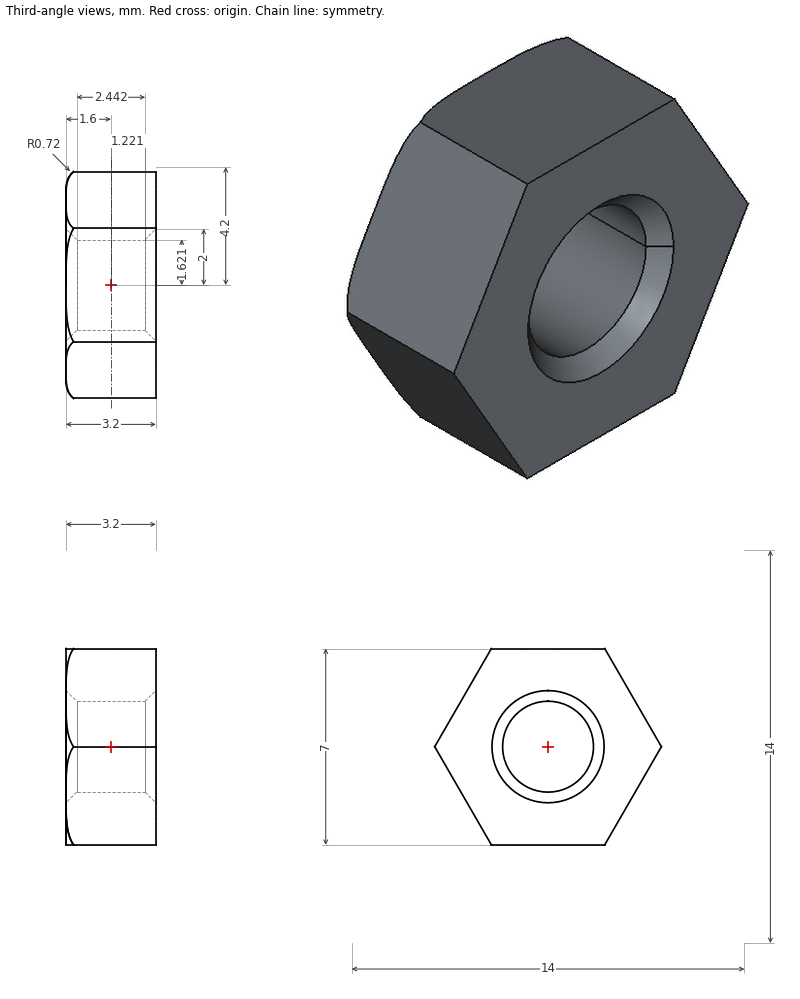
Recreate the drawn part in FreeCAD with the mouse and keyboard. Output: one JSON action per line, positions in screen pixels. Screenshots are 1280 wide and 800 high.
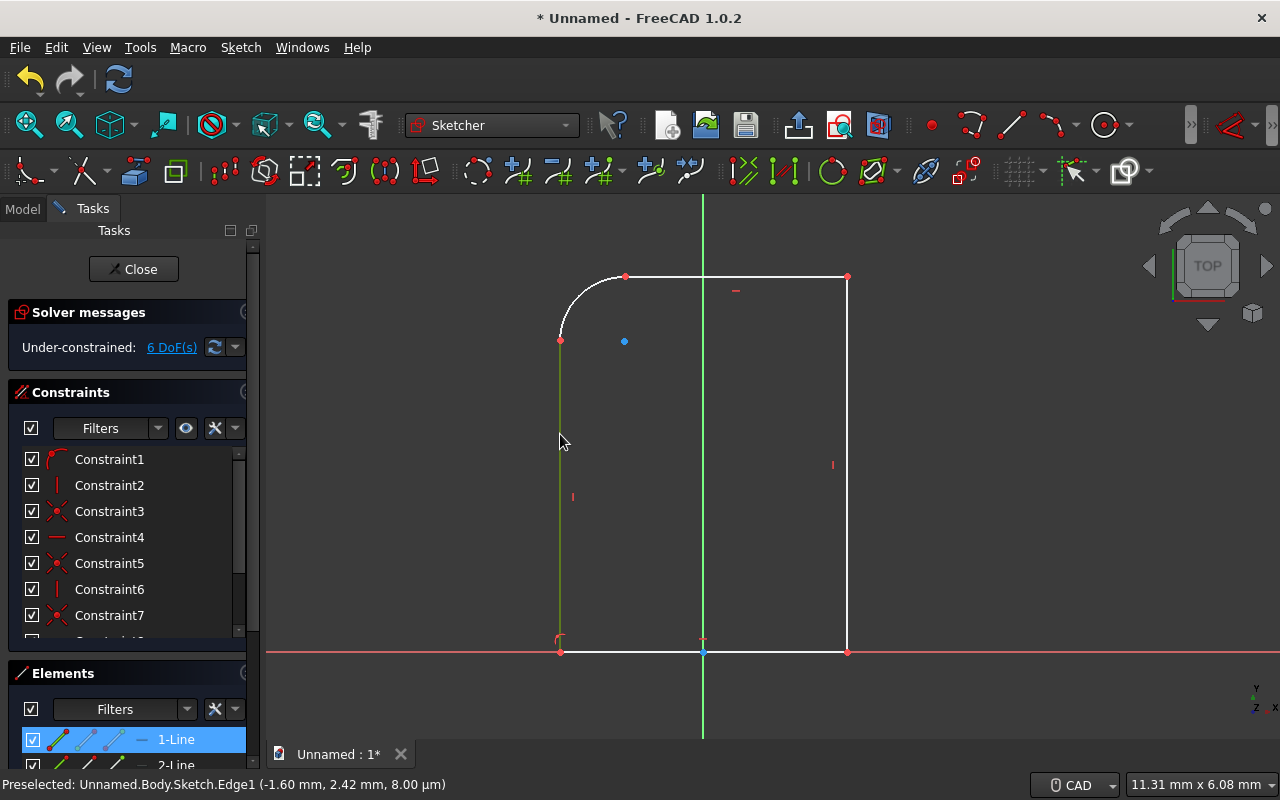
{"action": "left_click", "coordinate": [596, 284]}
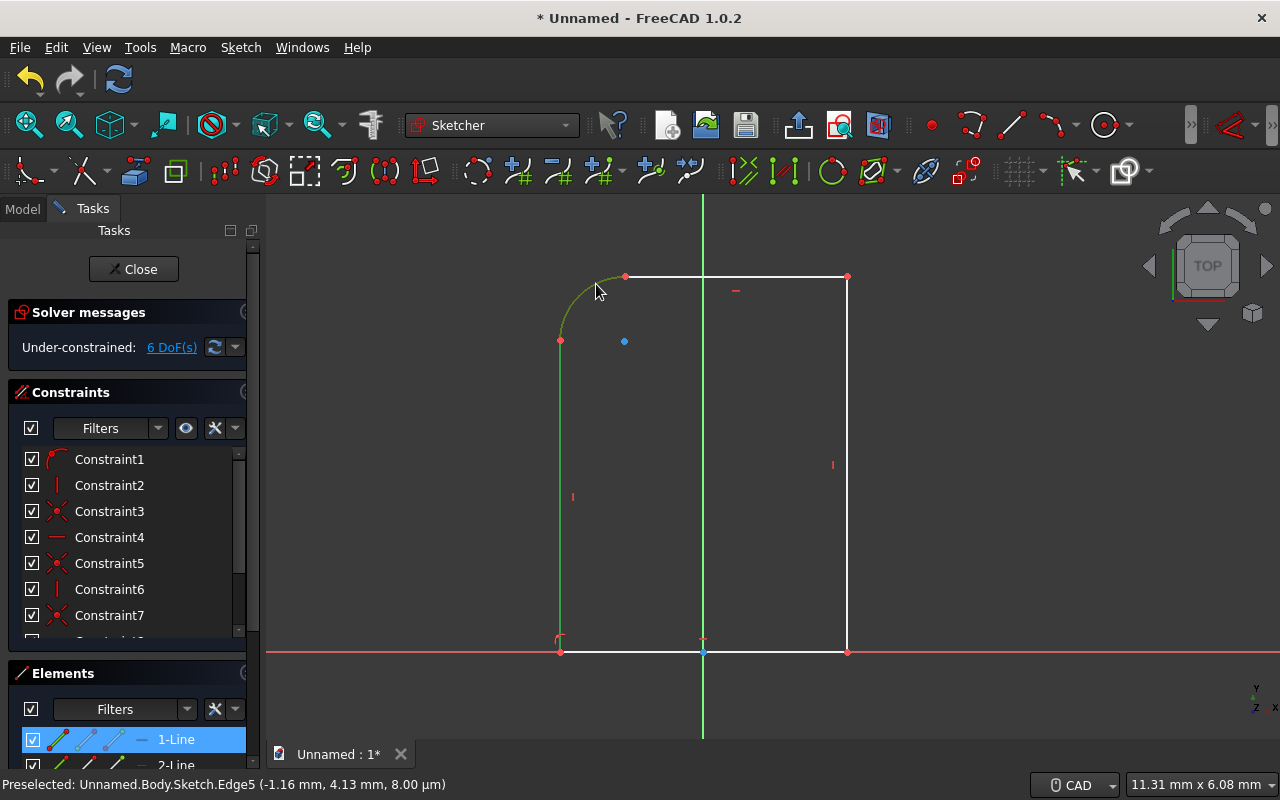
{"action": "key", "text": "t"}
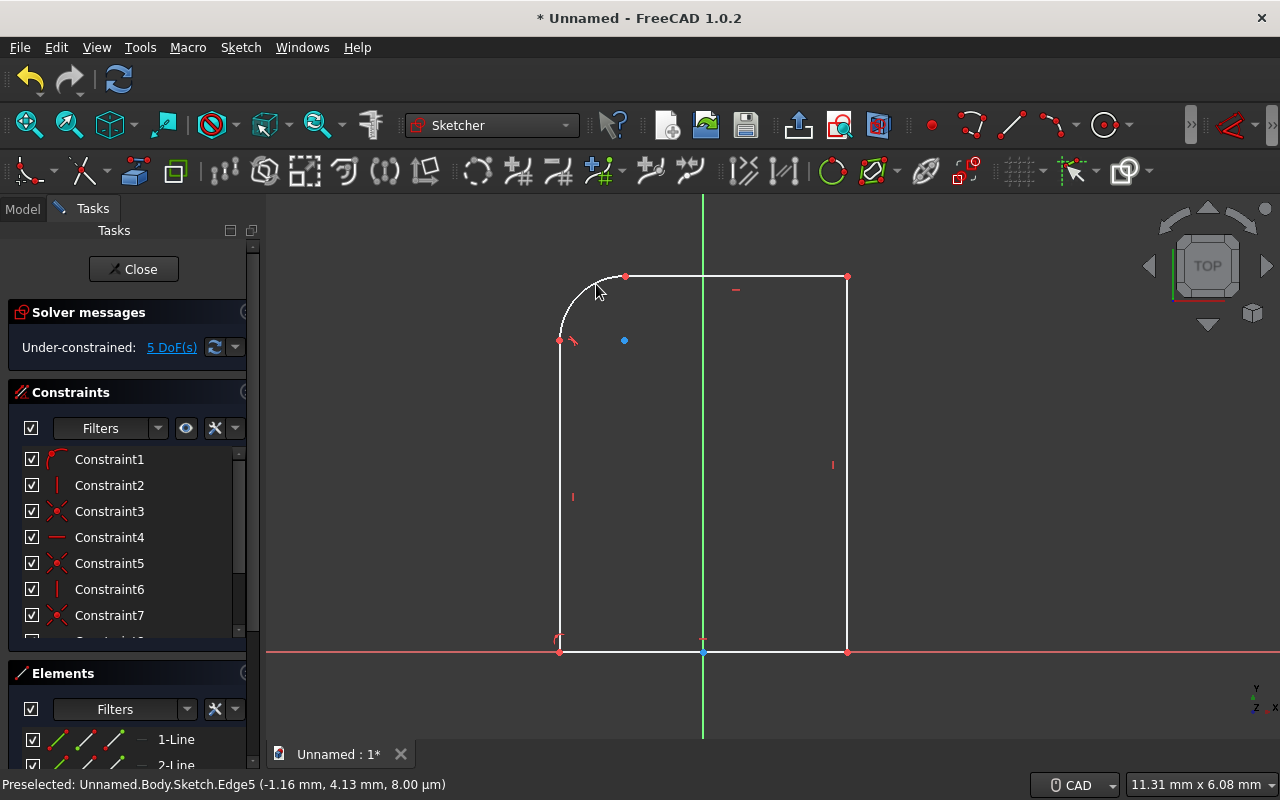
{"action": "left_click", "coordinate": [780, 276]}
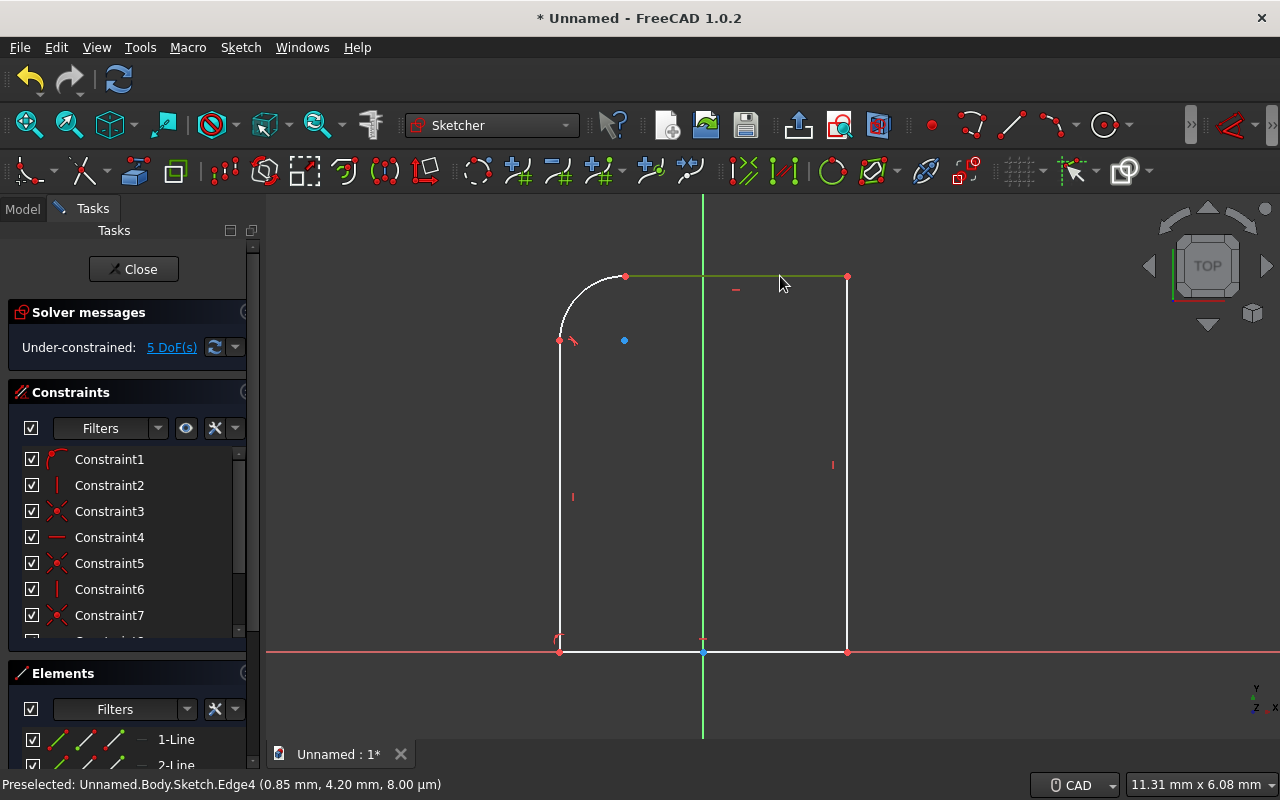
{"action": "left_click", "coordinate": [595, 283]}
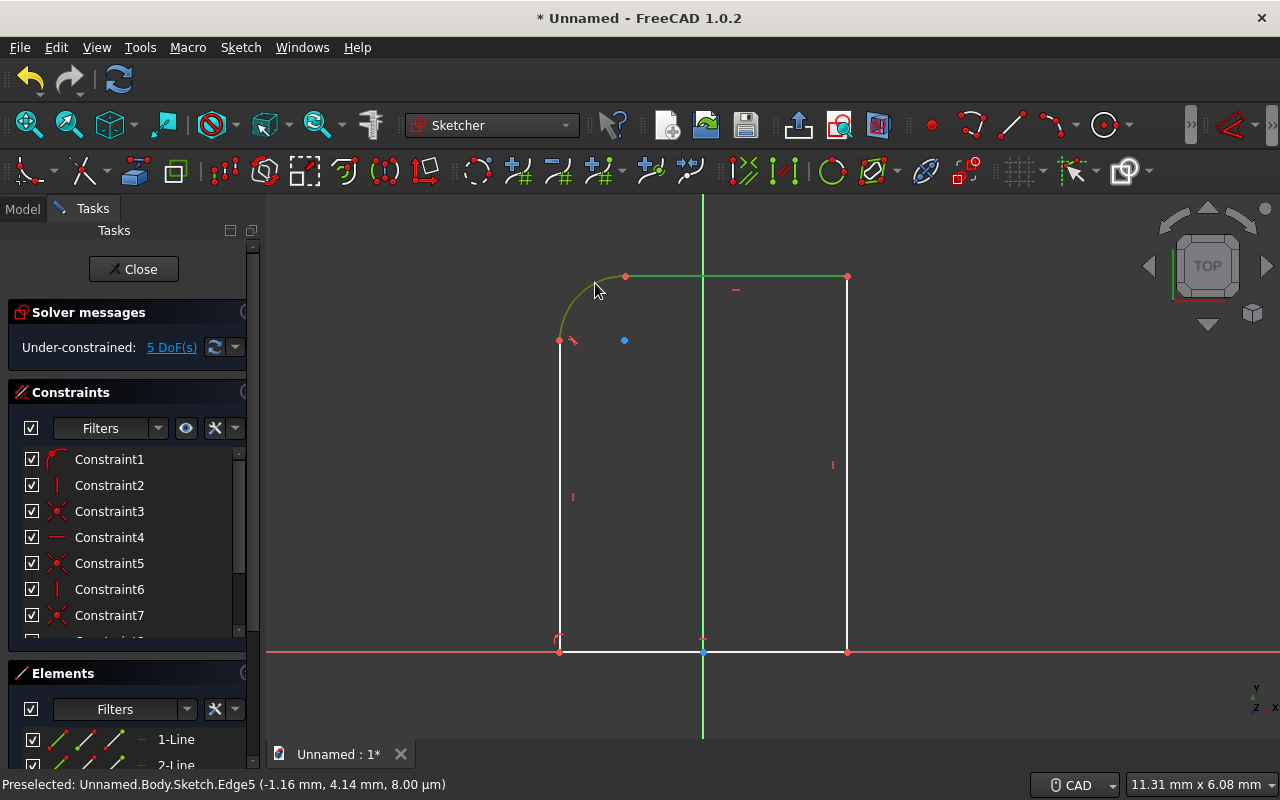
{"action": "key", "text": "t"}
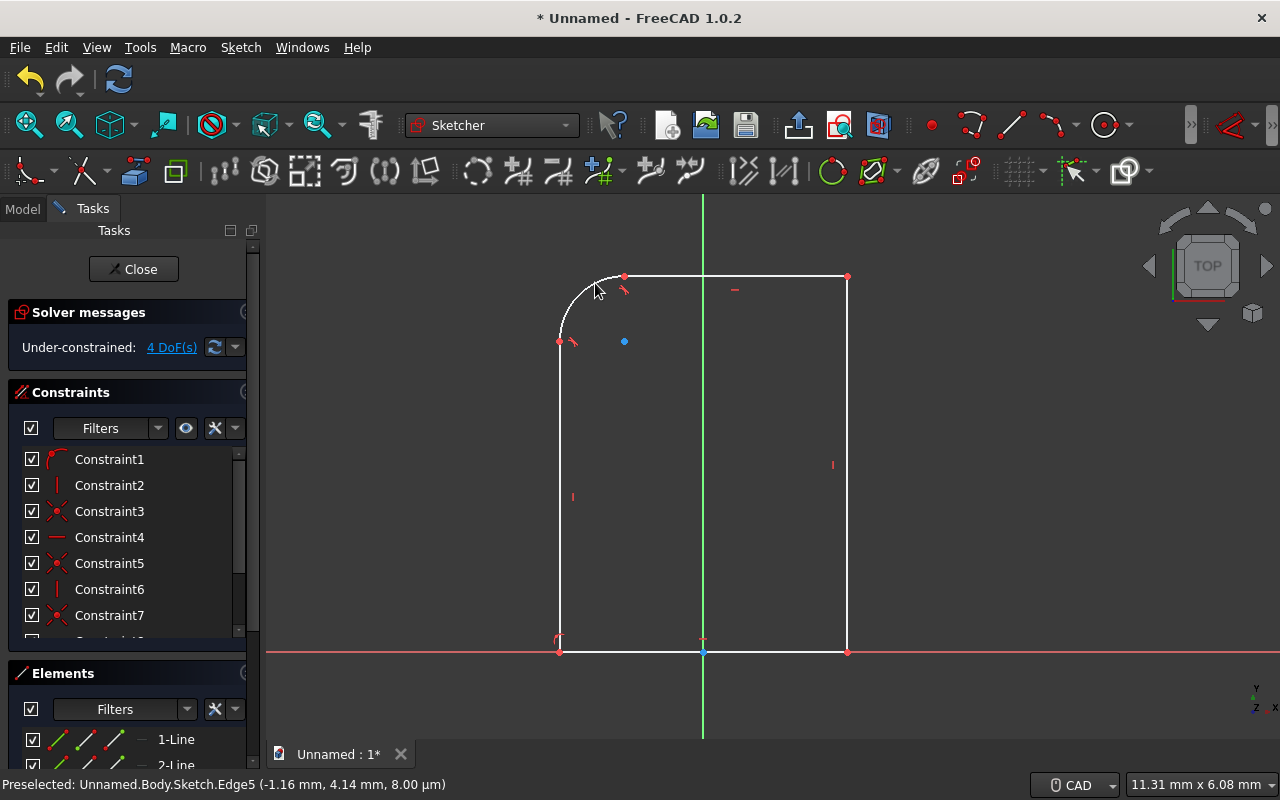
{"action": "key", "text": "d"}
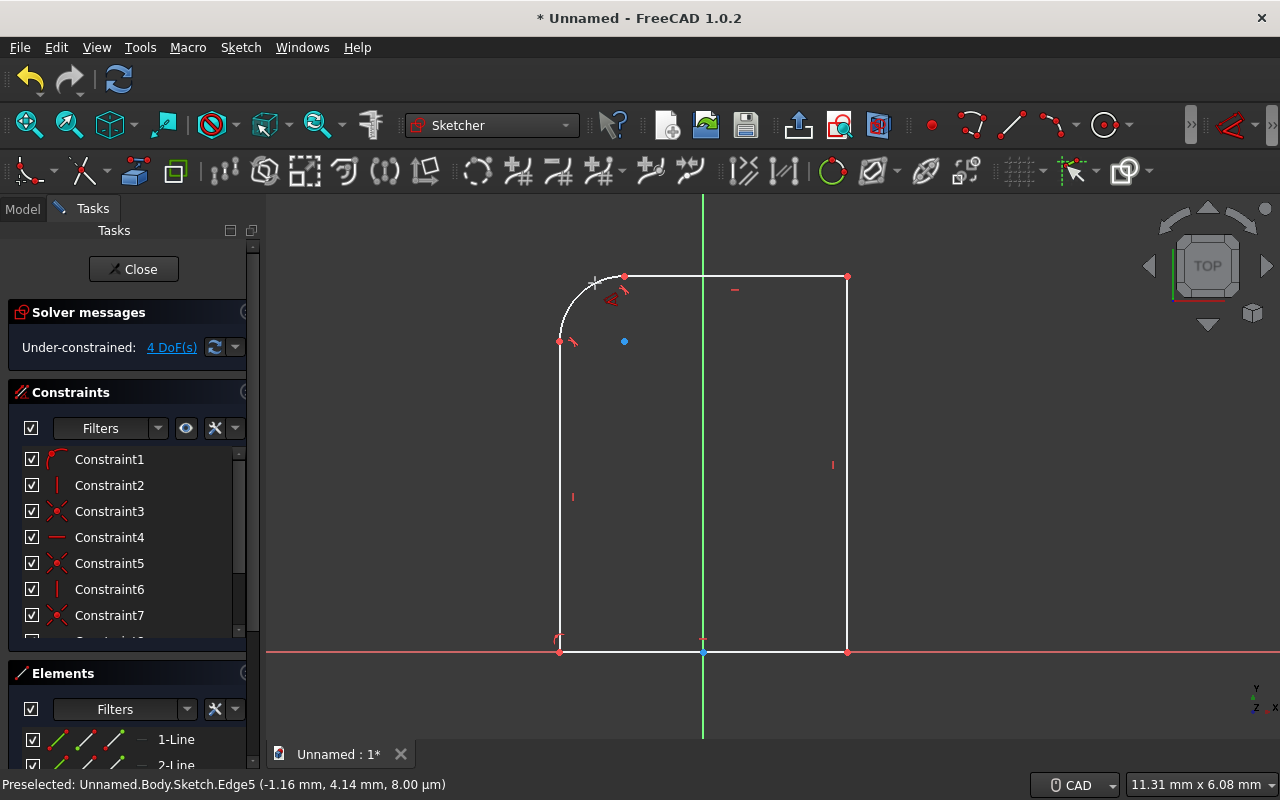
{"action": "left_click", "coordinate": [595, 283]}
{"action": "left_click", "coordinate": [580, 255]}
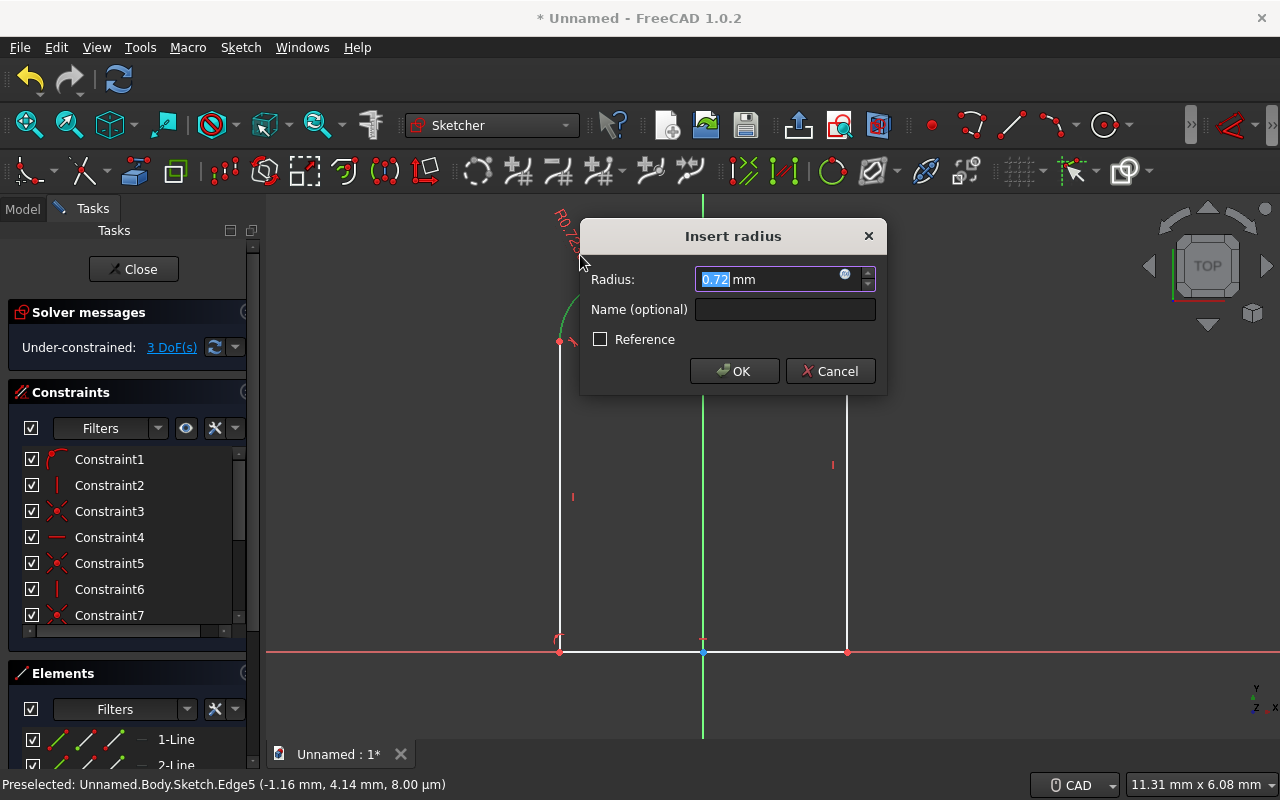
{"action": "type", "text": "0.72"}
{"action": "key", "text": "Return"}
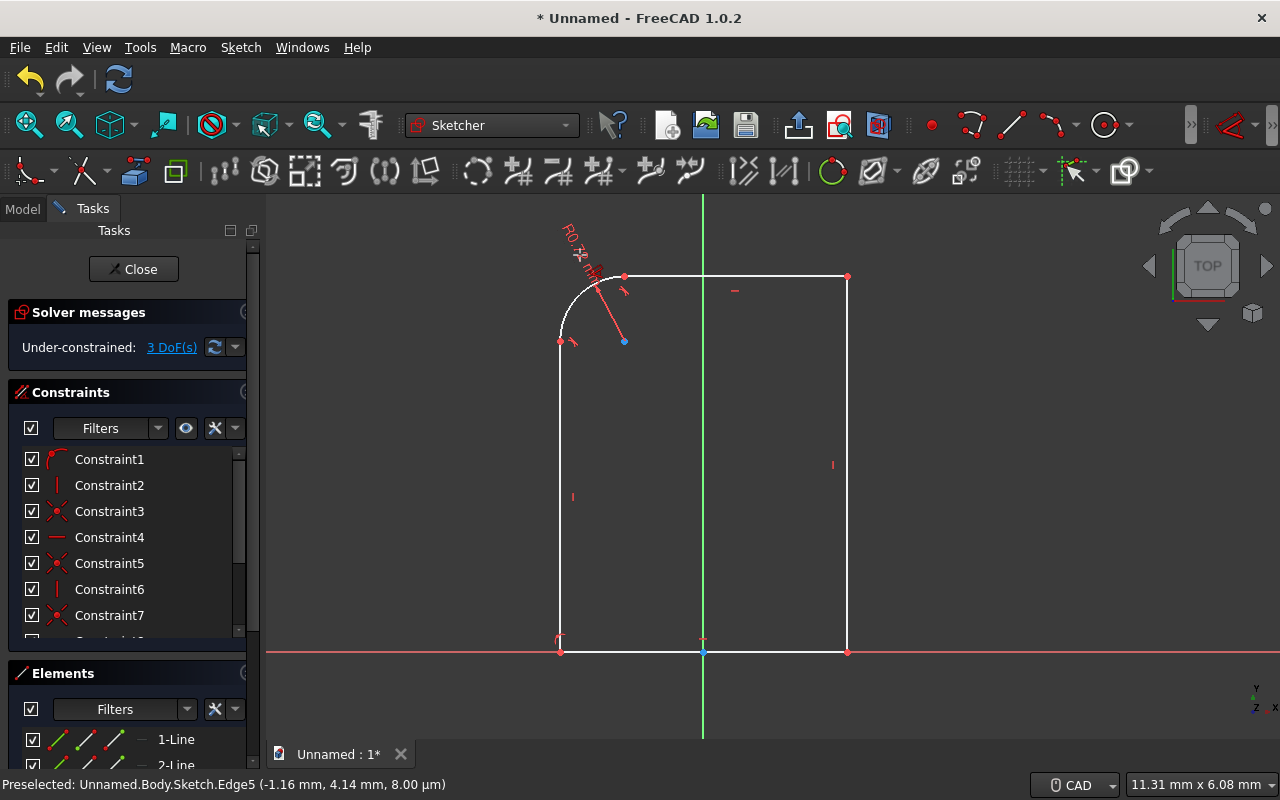
{"action": "left_click", "coordinate": [646, 652]}
{"action": "left_click", "coordinate": [638, 686]}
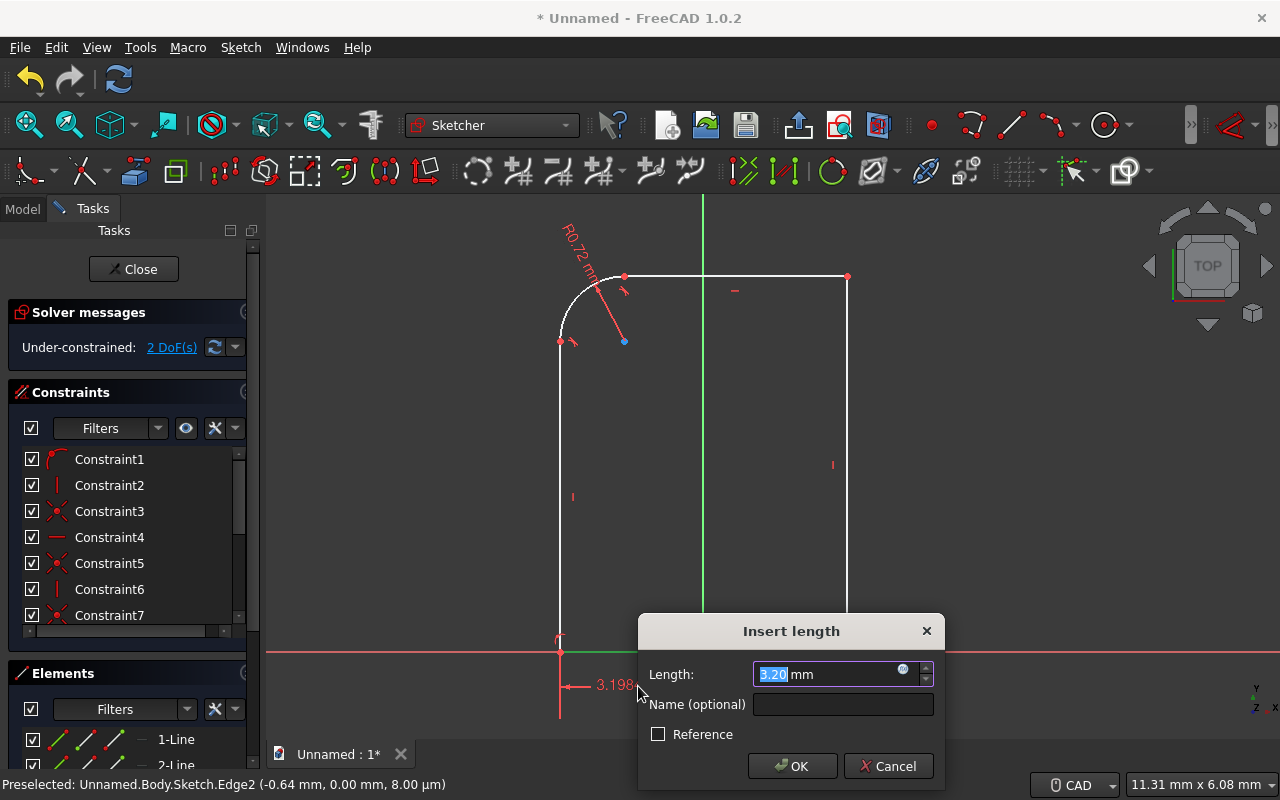
{"action": "type", "text": "3.2"}
{"action": "key", "text": "Return"}